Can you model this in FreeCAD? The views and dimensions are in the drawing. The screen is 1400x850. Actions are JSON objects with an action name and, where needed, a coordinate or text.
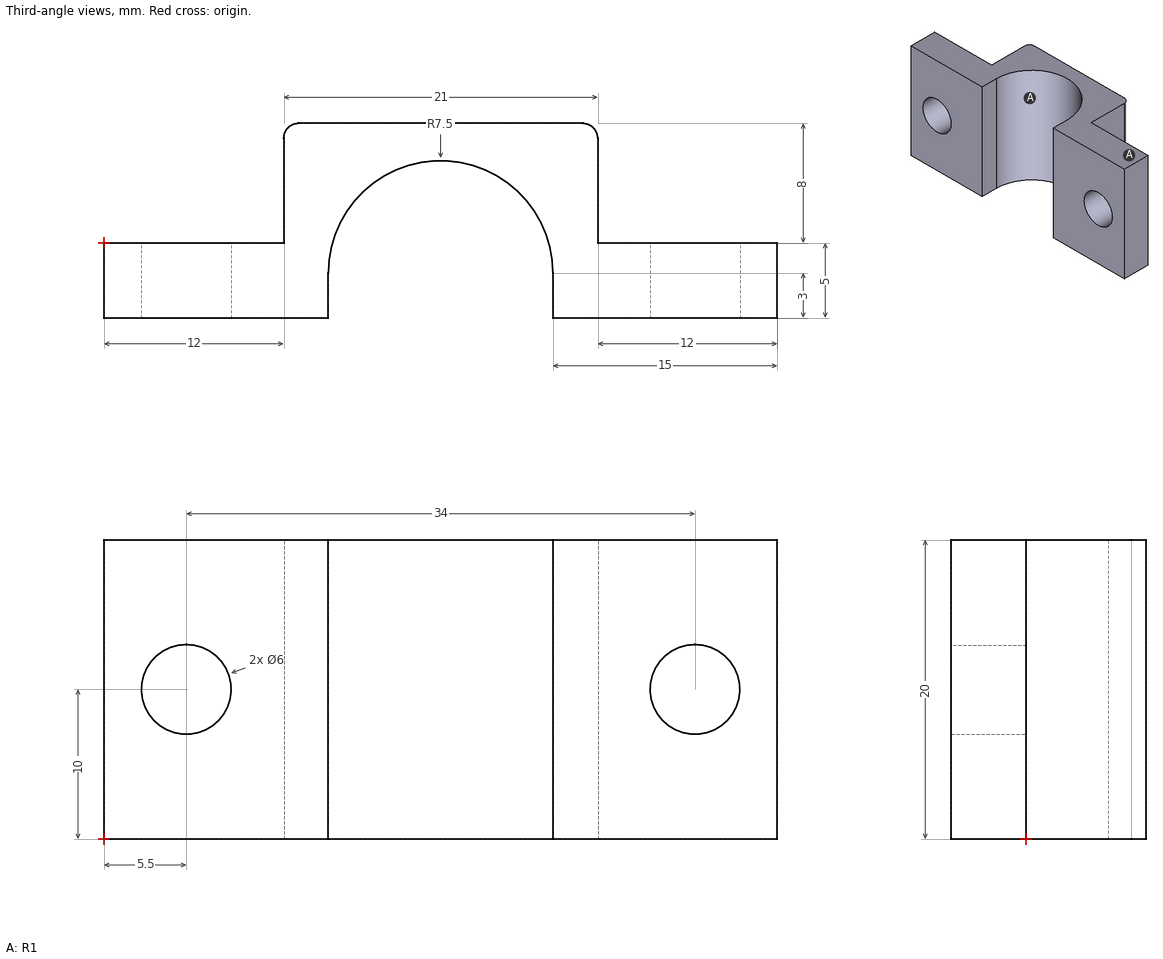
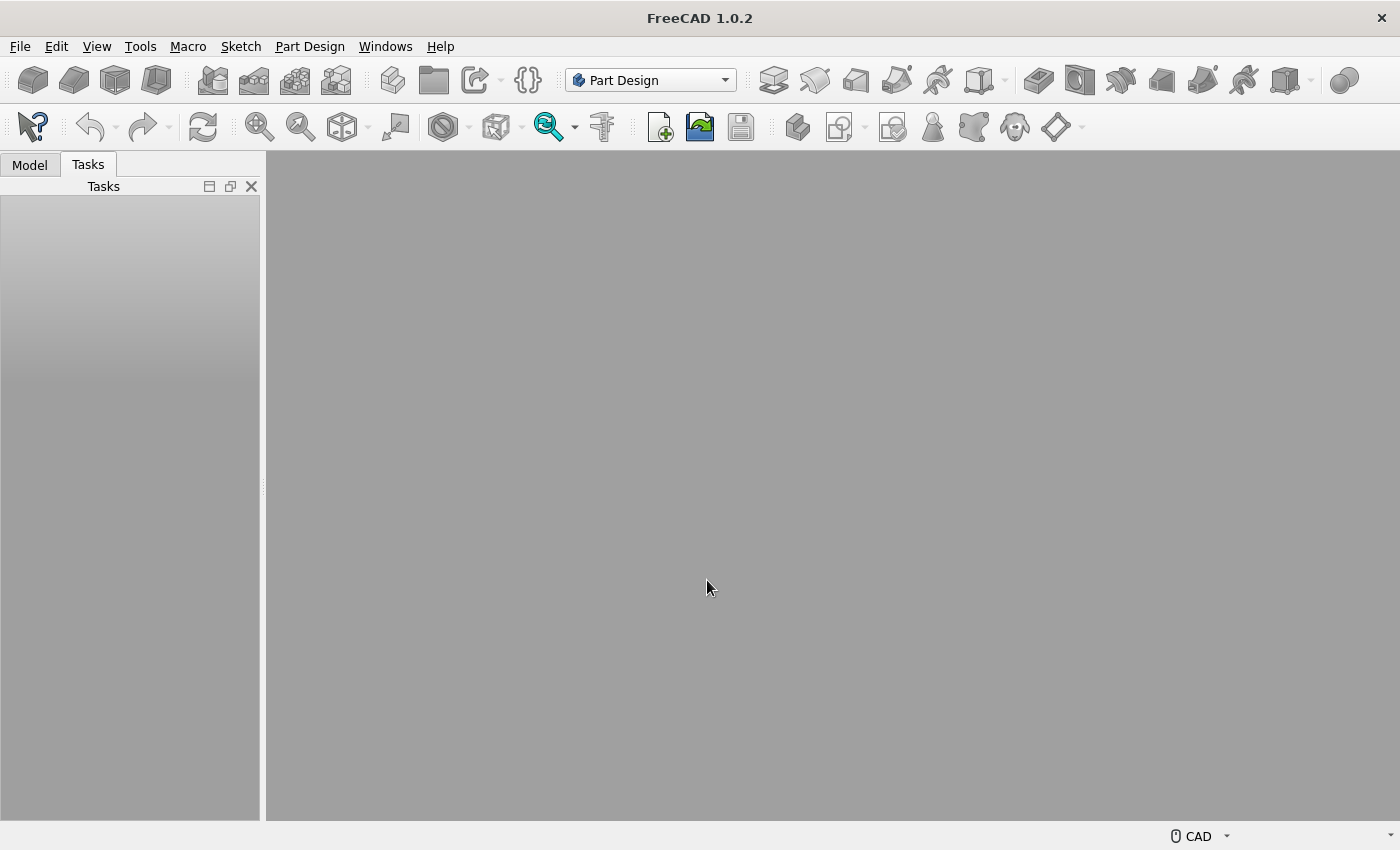
{"action": "key", "text": "ctrl+n"}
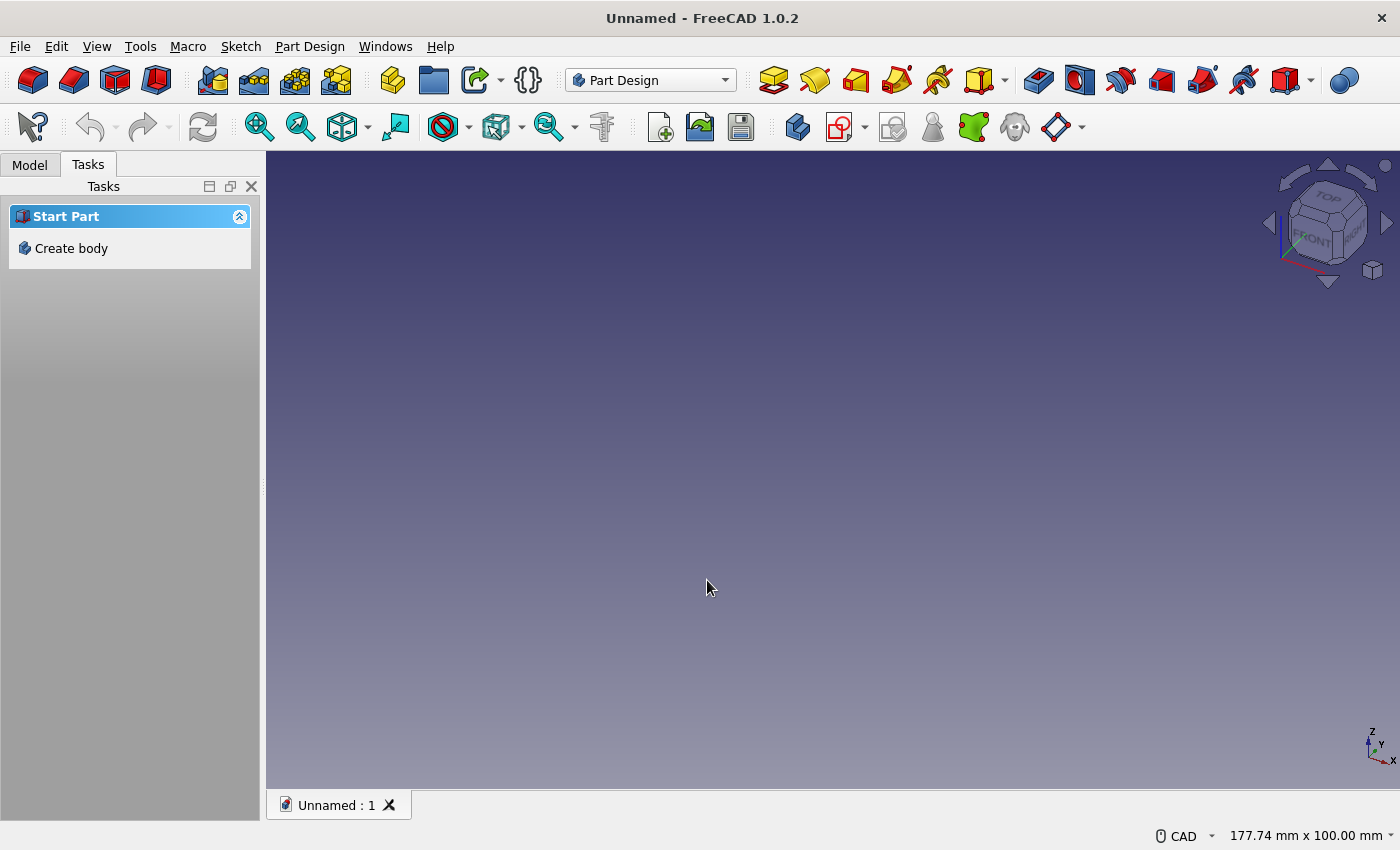
{"action": "left_click", "coordinate": [838, 128]}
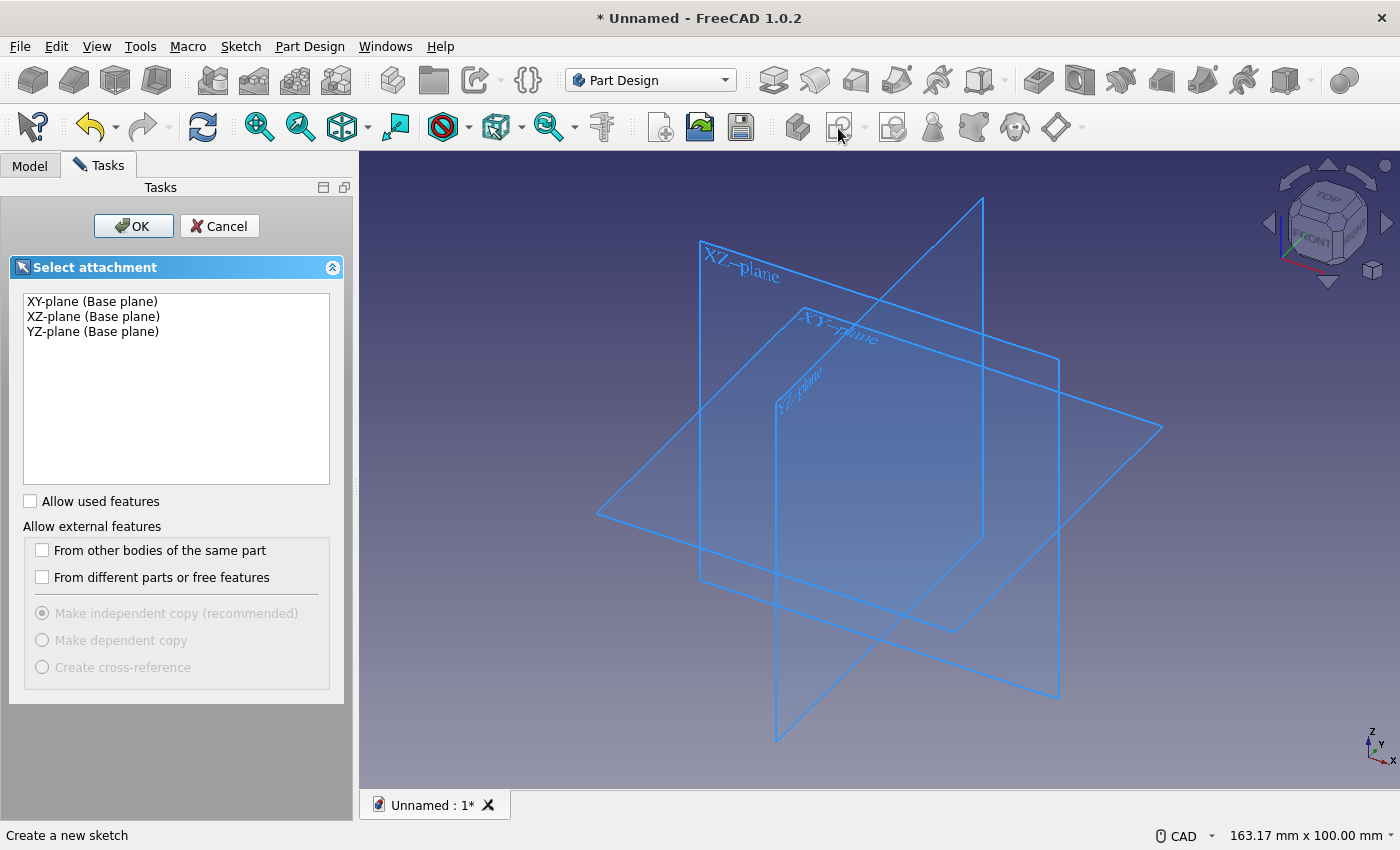
{"action": "left_click", "coordinate": [84, 302]}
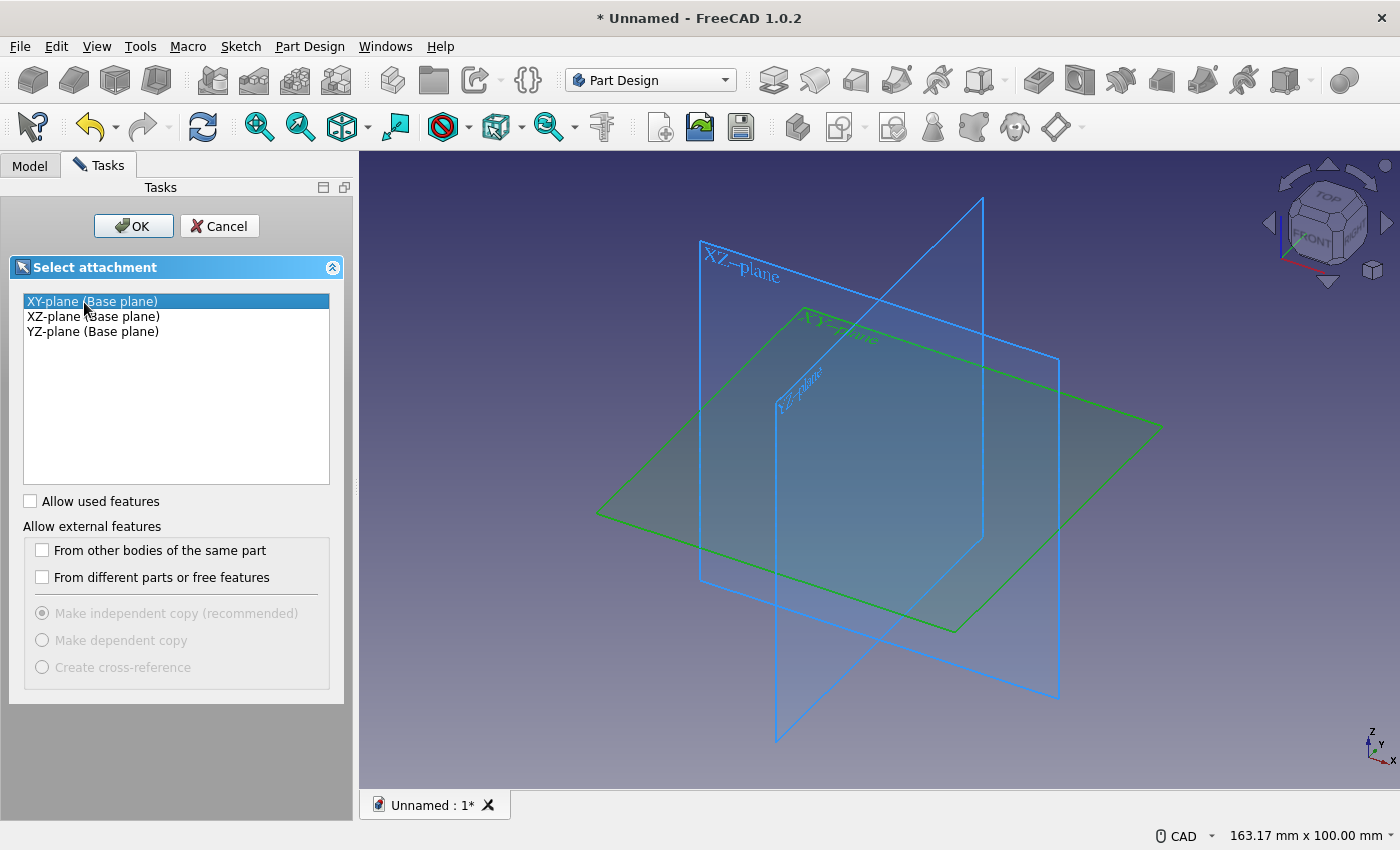
{"action": "left_click", "coordinate": [134, 226]}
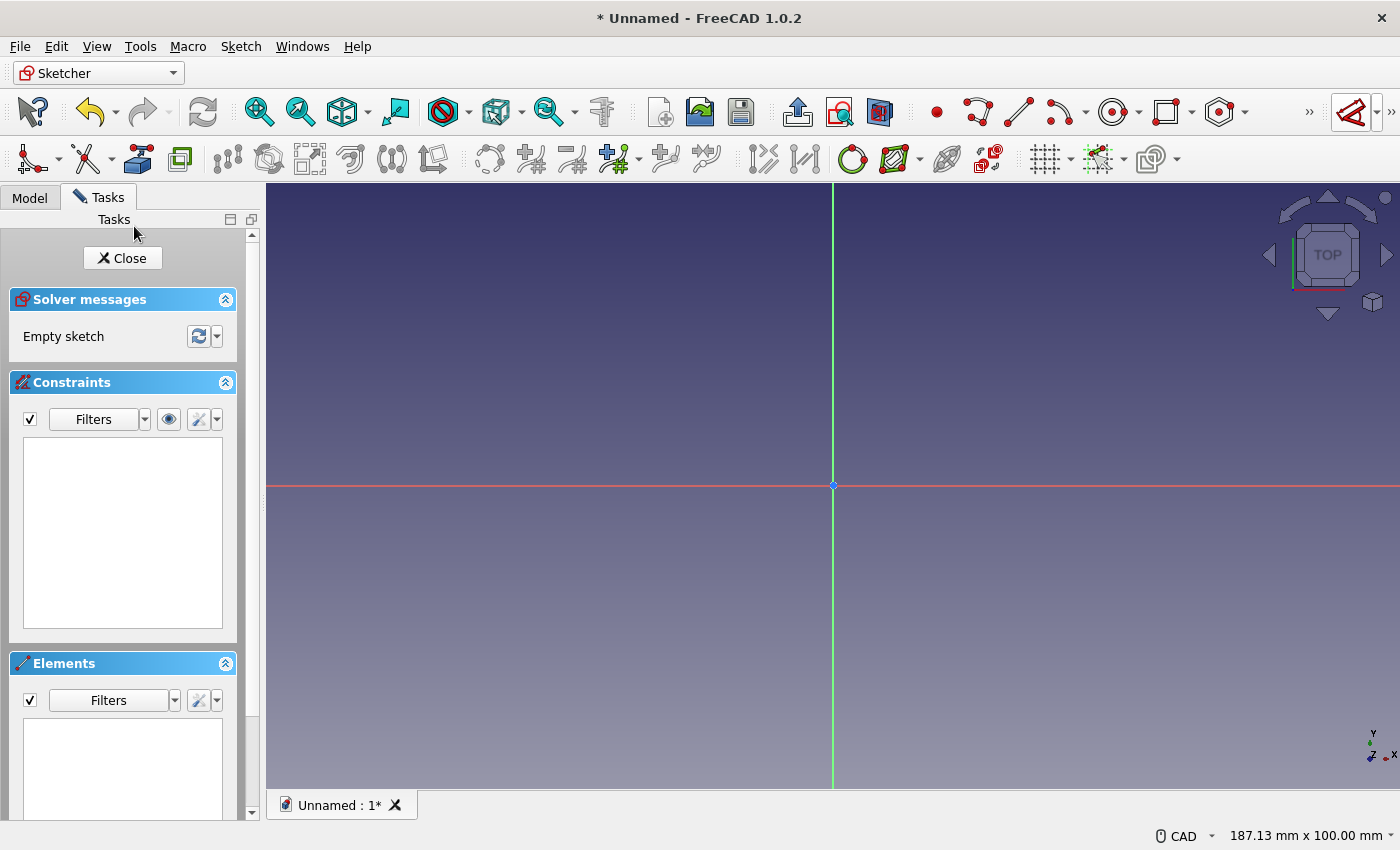
{"action": "scroll", "coordinate": [1137, 469], "scroll_direction": "up", "scroll_amount": 4}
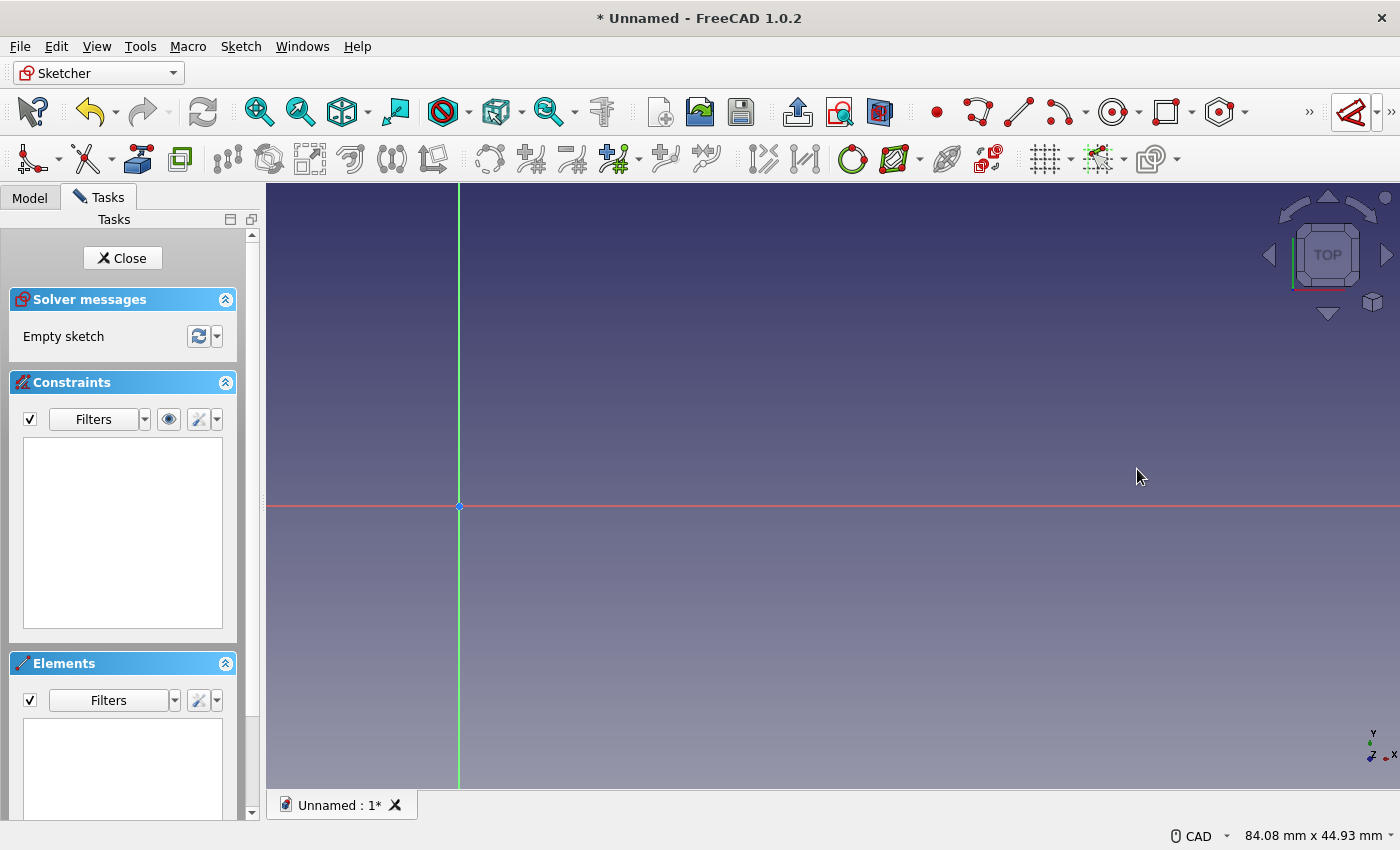
{"action": "left_click", "coordinate": [978, 112]}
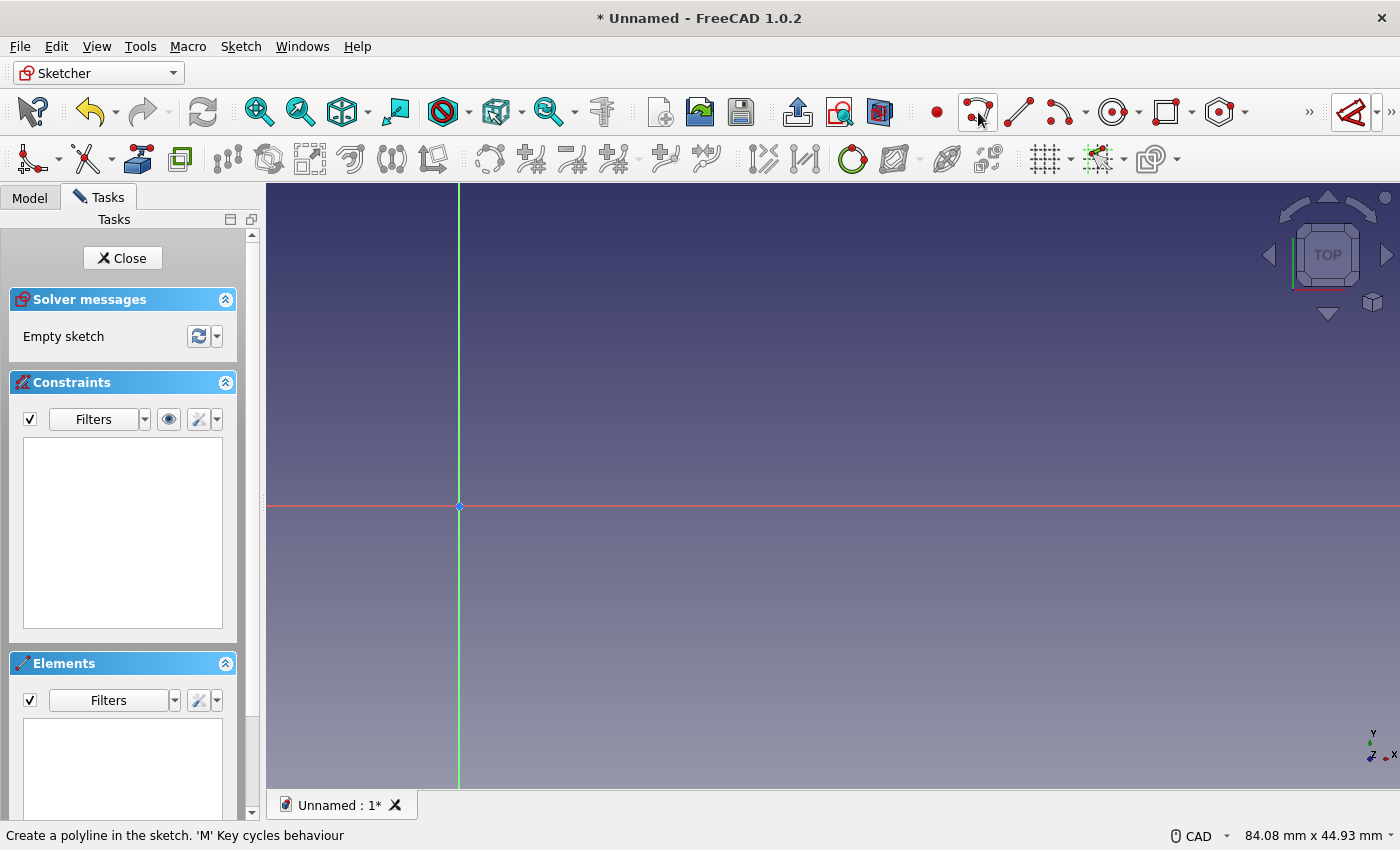
{"action": "left_click", "coordinate": [864, 533]}
{"action": "left_click", "coordinate": [864, 574]}
{"action": "left_click", "coordinate": [1066, 574]}
{"action": "left_click", "coordinate": [1066, 506]}
{"action": "left_click", "coordinate": [905, 497]}
{"action": "left_click", "coordinate": [905, 398]}
{"action": "left_click", "coordinate": [621, 398]}
{"action": "left_click", "coordinate": [621, 506]}
{"action": "left_click", "coordinate": [459, 506]}
{"action": "left_click", "coordinate": [468, 574]}
{"action": "left_click", "coordinate": [662, 574]}
{"action": "left_click", "coordinate": [662, 533]}
{"action": "right_click", "coordinate": [662, 533]}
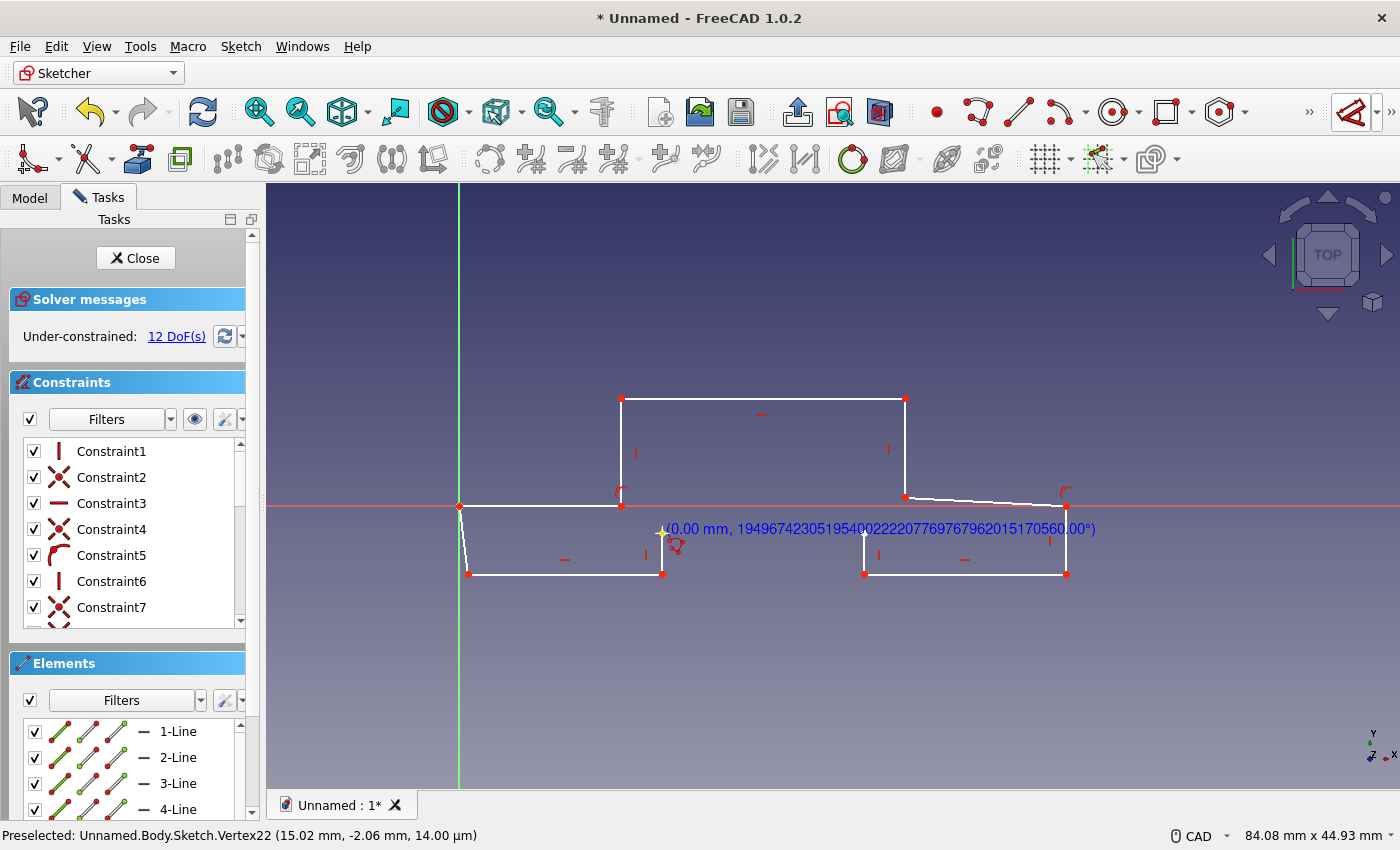
{"action": "key", "text": "g 3 a"}